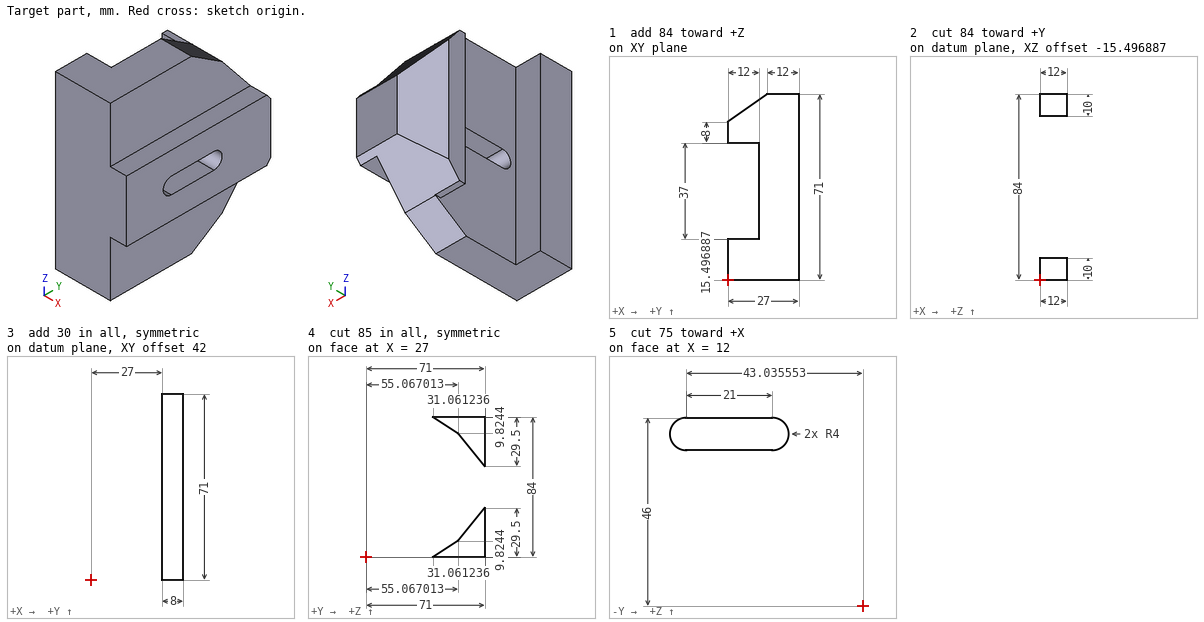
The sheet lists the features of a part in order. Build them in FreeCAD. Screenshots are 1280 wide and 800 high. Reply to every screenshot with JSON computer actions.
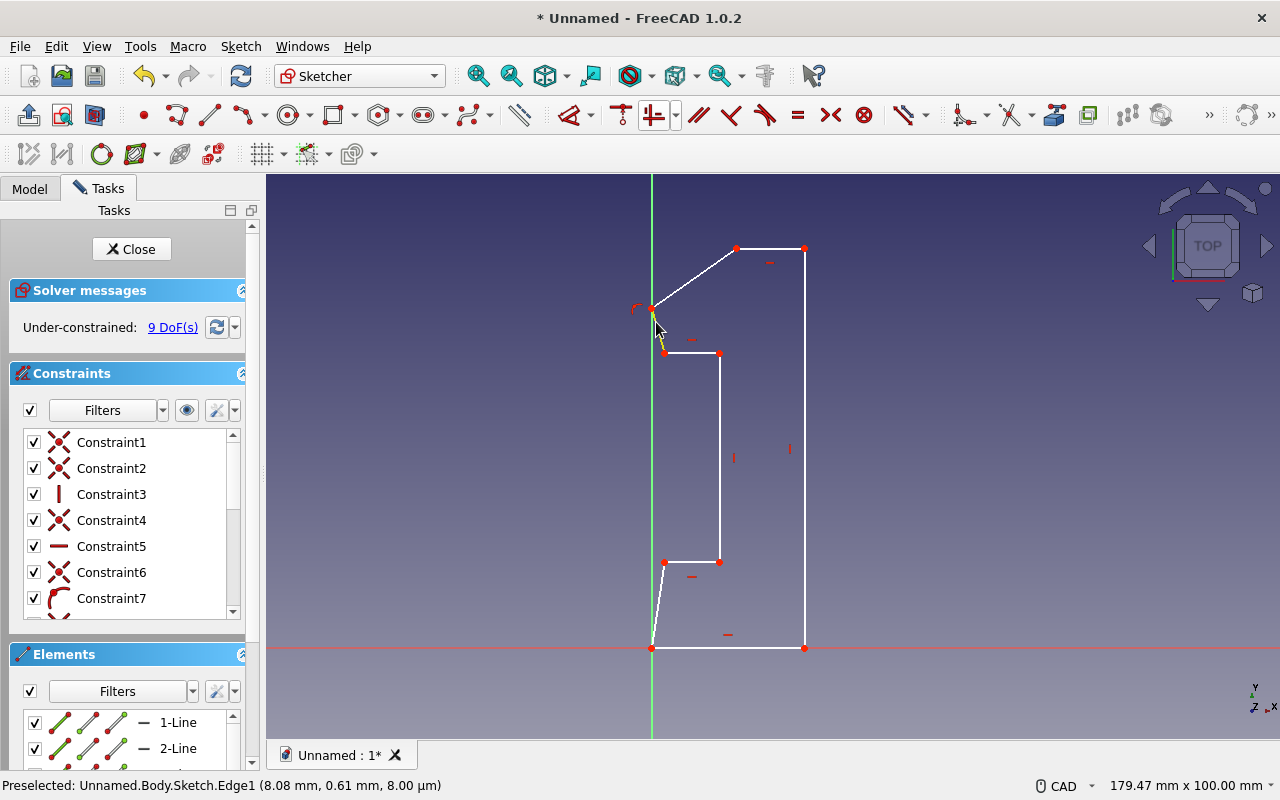
{"action": "left_click", "coordinate": [656, 322]}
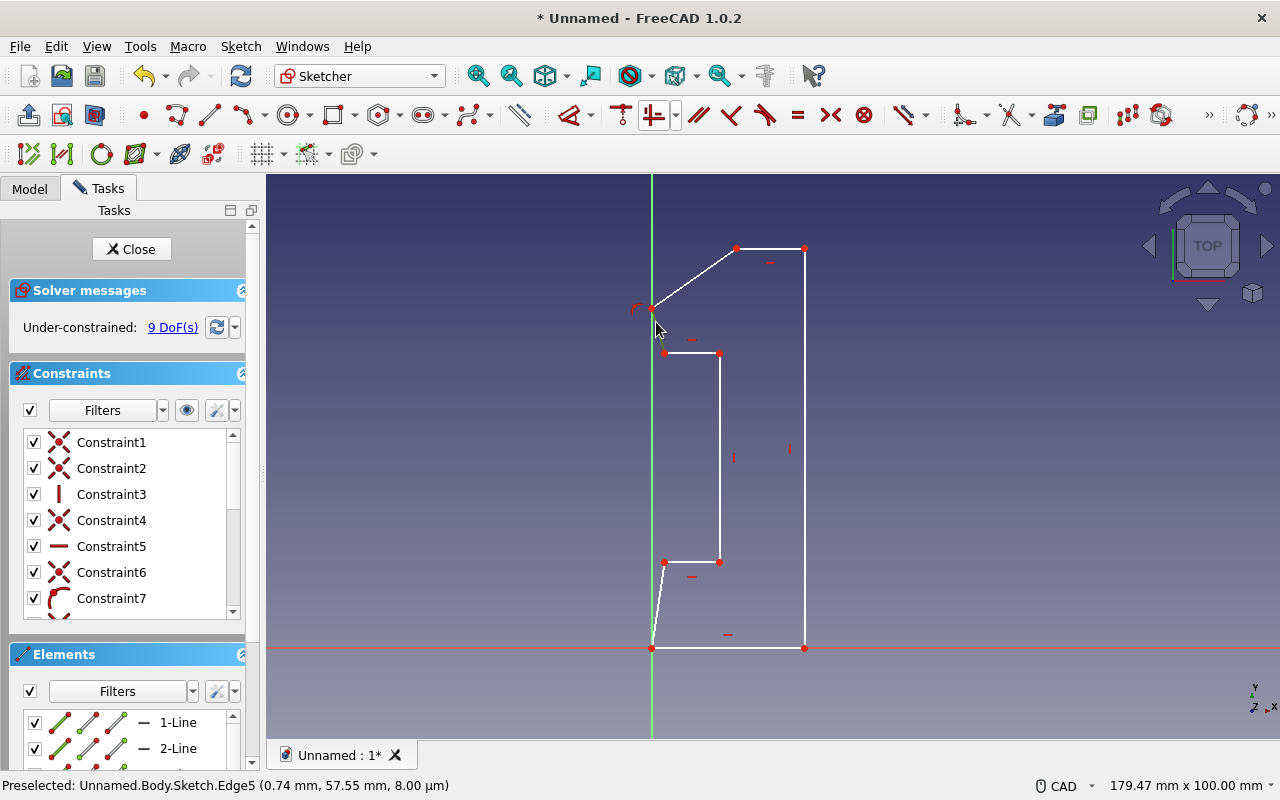
{"action": "key", "text": "v"}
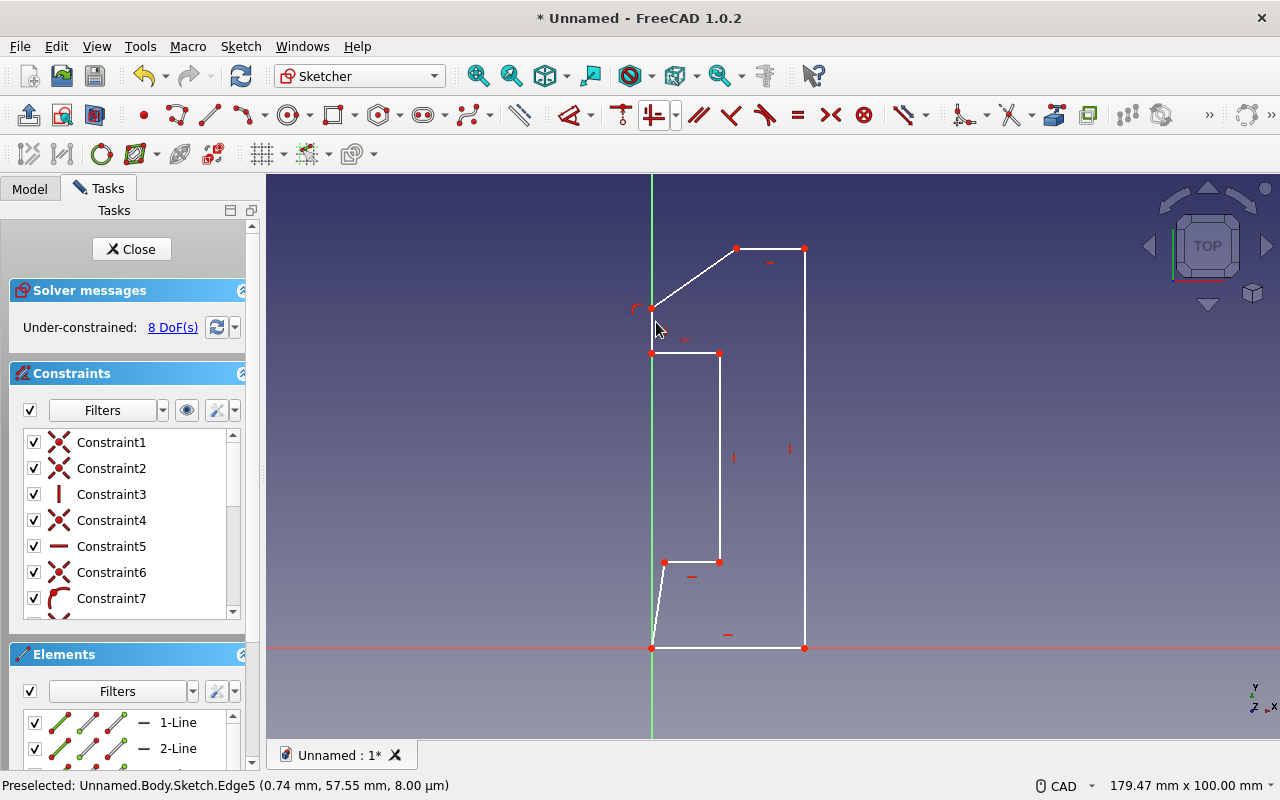
{"action": "scroll", "coordinate": [661, 588], "scroll_direction": "up", "scroll_amount": 3}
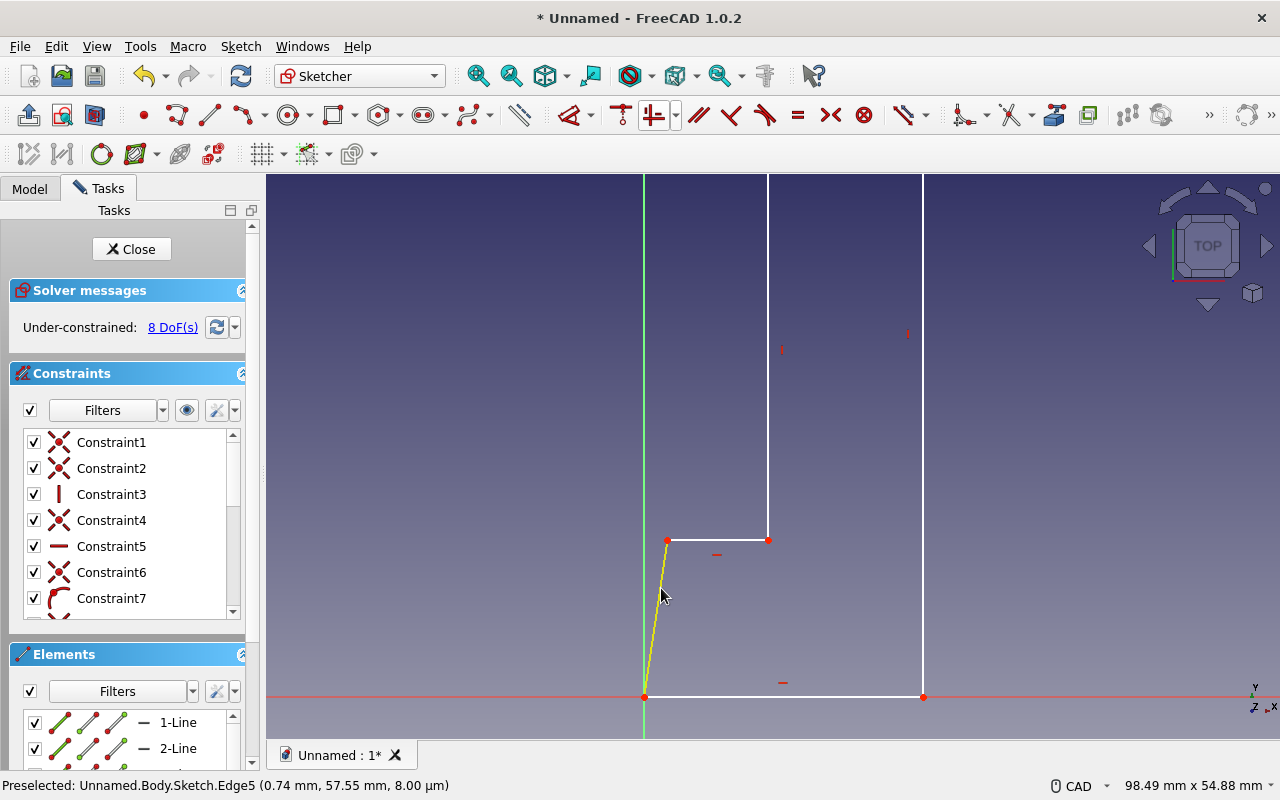
{"action": "left_click", "coordinate": [660, 587]}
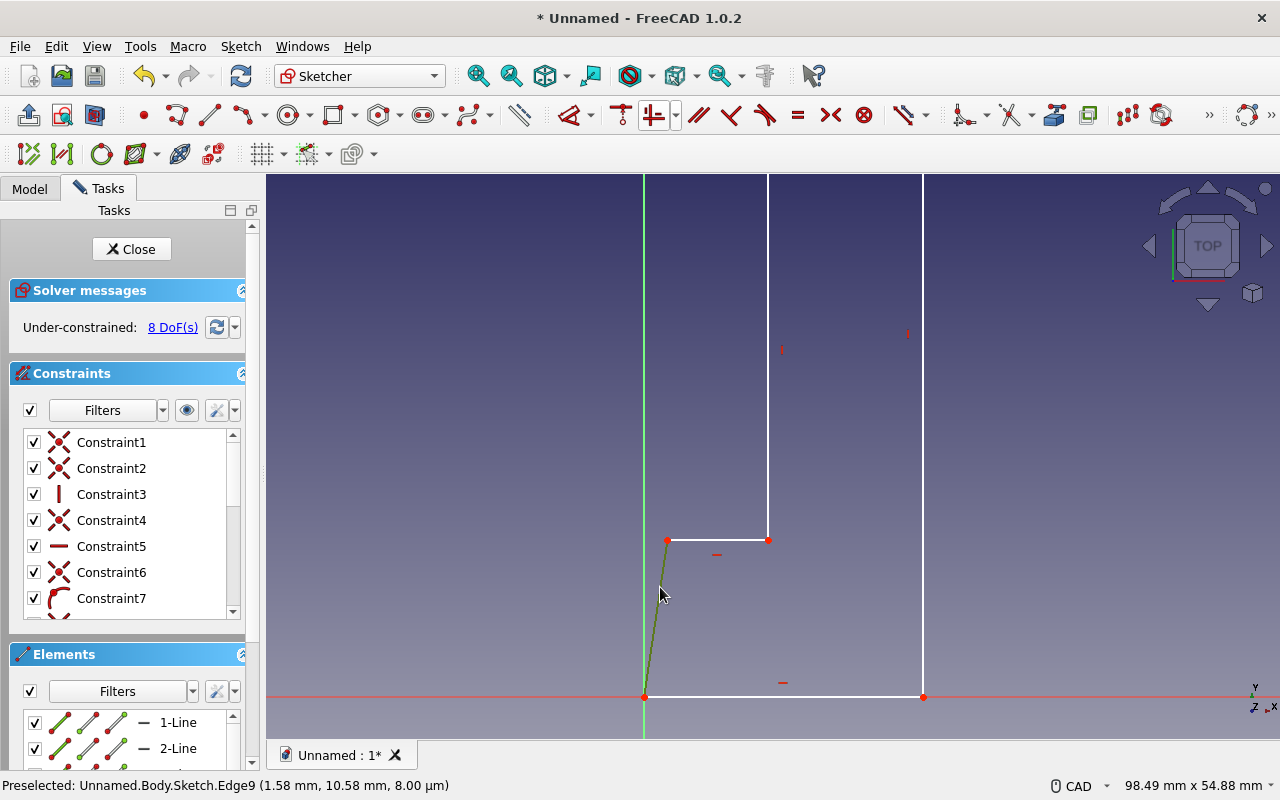
{"action": "left_click", "coordinate": [676, 116]}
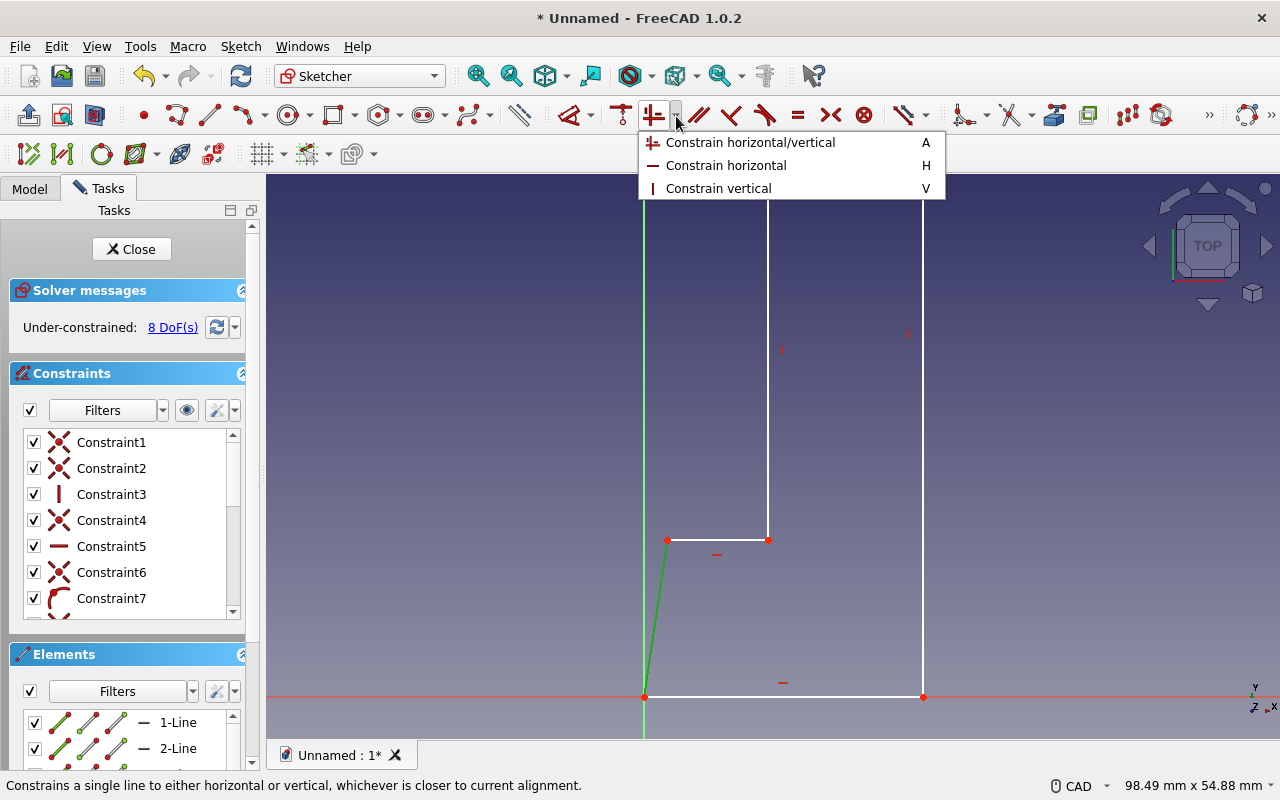
{"action": "left_click", "coordinate": [792, 188]}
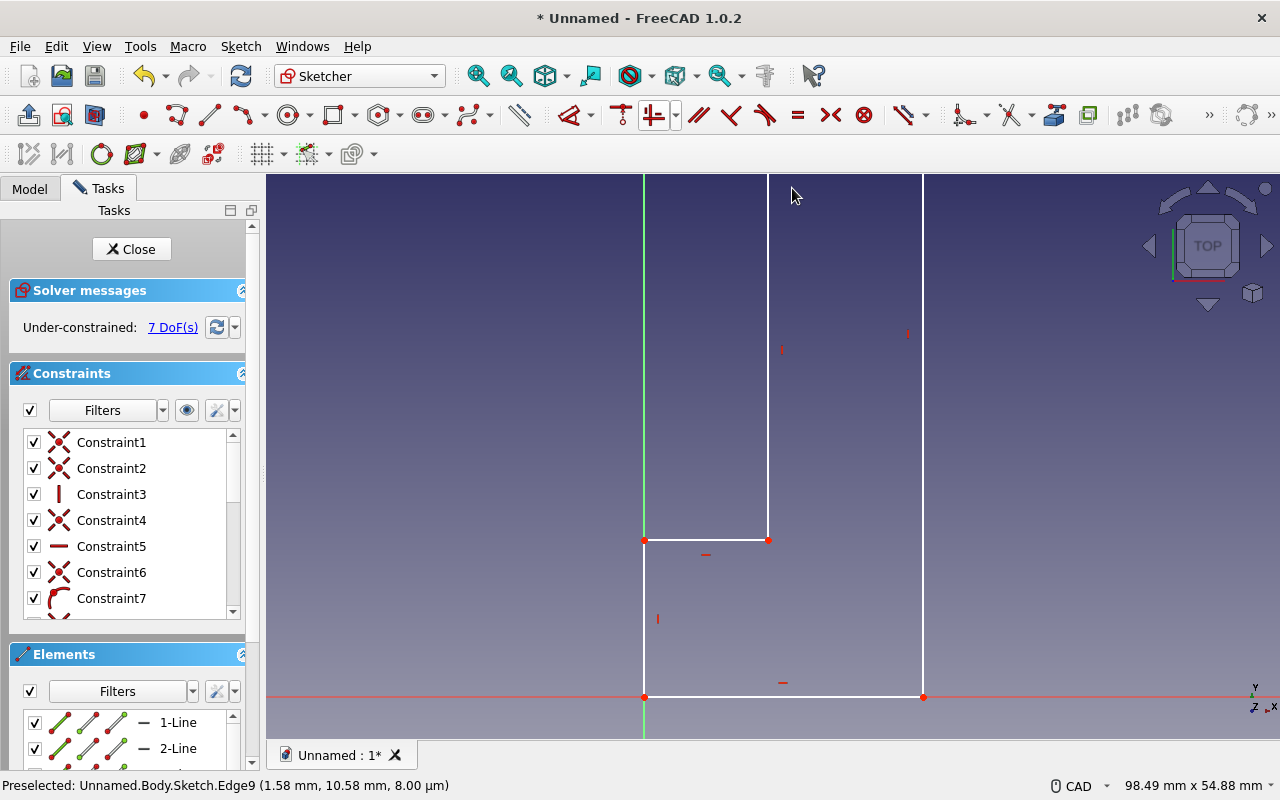
{"action": "scroll", "coordinate": [640, 558], "scroll_direction": "down", "scroll_amount": 4}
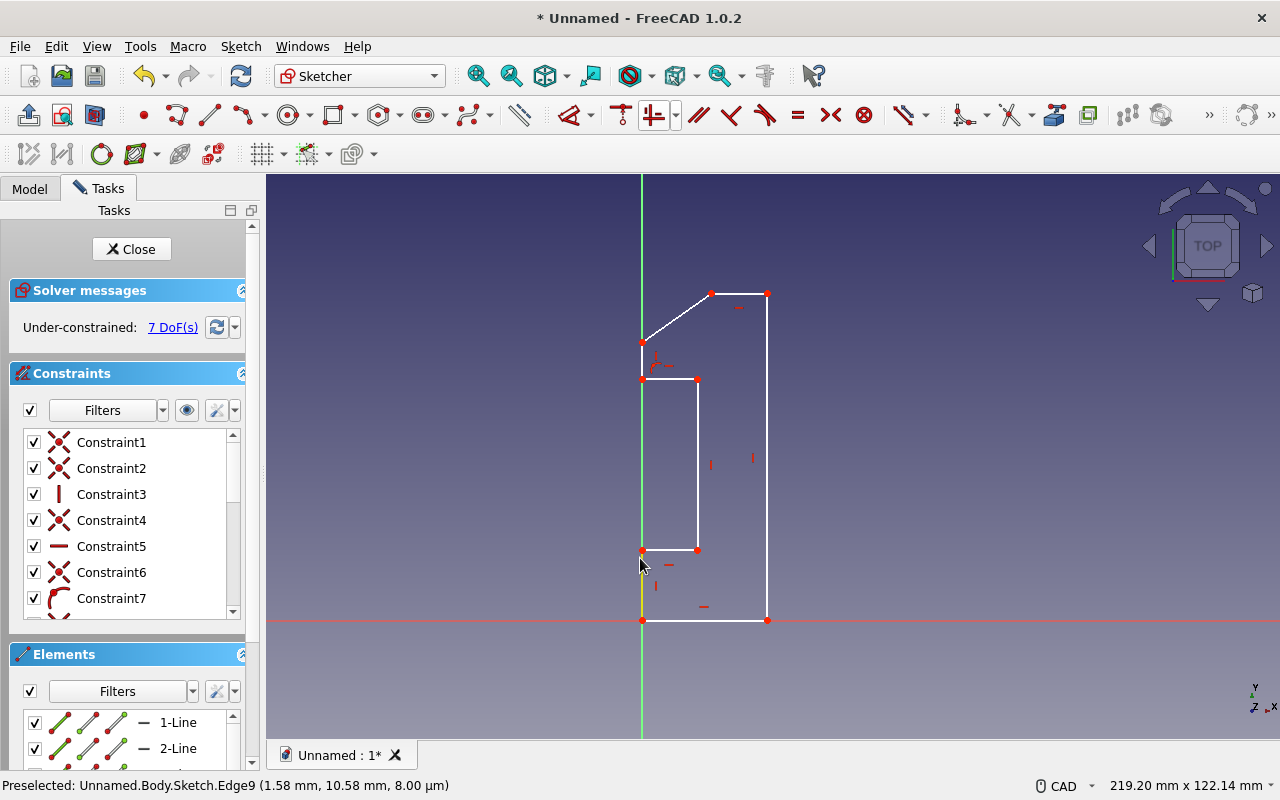
{"action": "scroll", "coordinate": [642, 354], "scroll_direction": "up", "scroll_amount": 2}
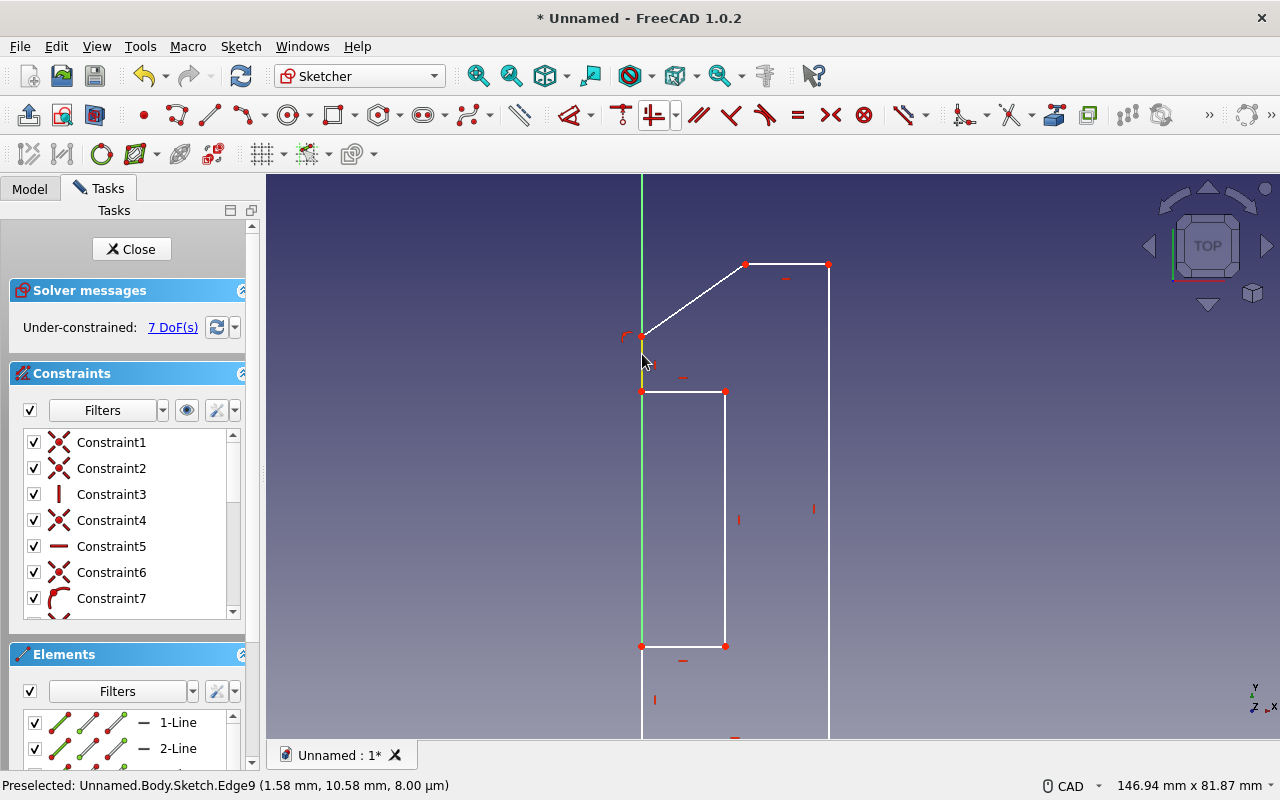
{"action": "left_click", "coordinate": [642, 353]}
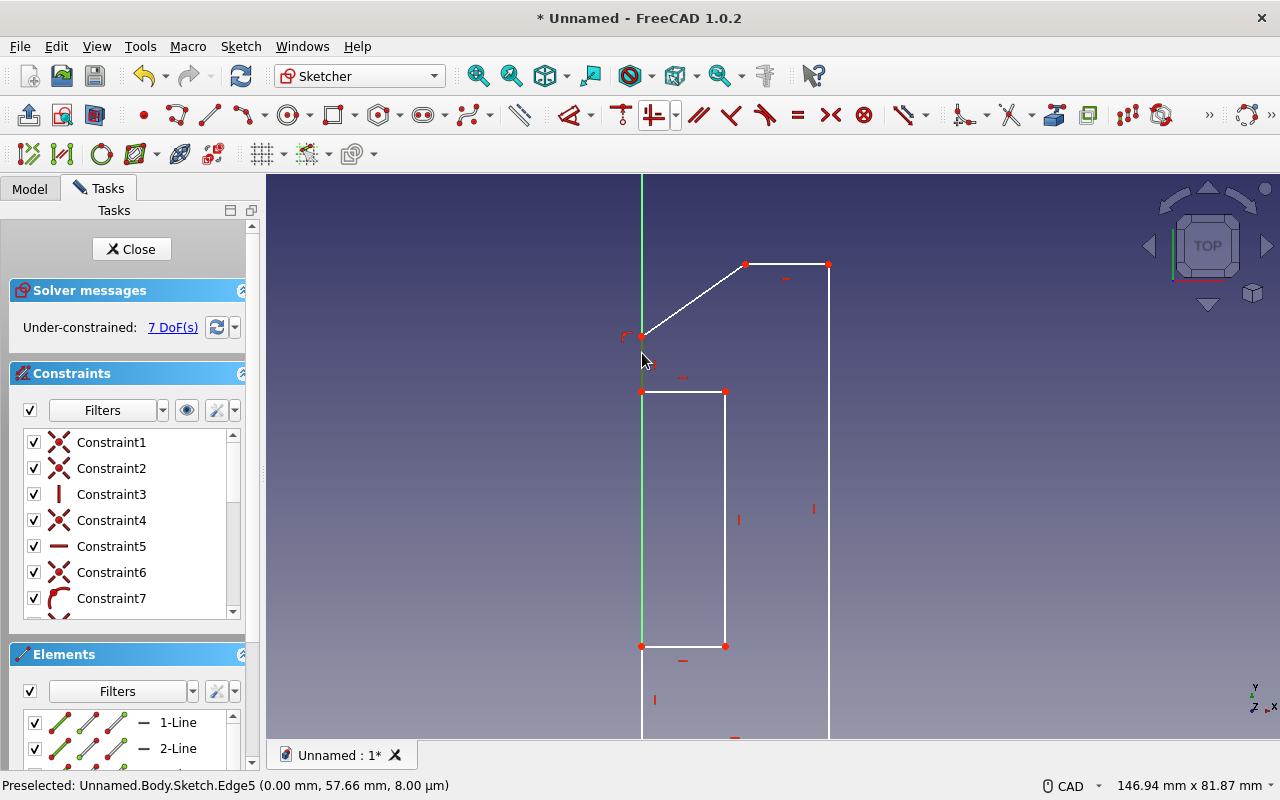
{"action": "key", "text": "i"}